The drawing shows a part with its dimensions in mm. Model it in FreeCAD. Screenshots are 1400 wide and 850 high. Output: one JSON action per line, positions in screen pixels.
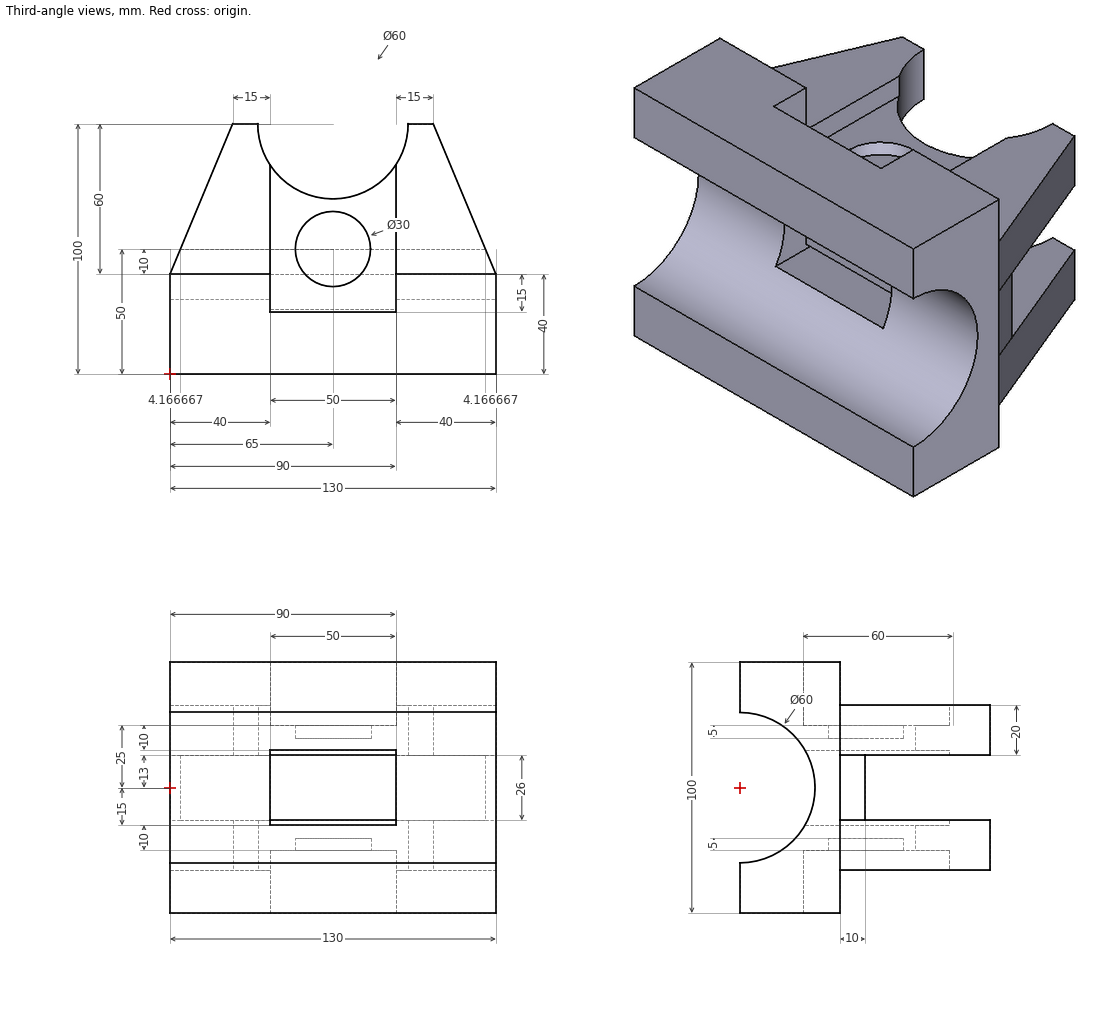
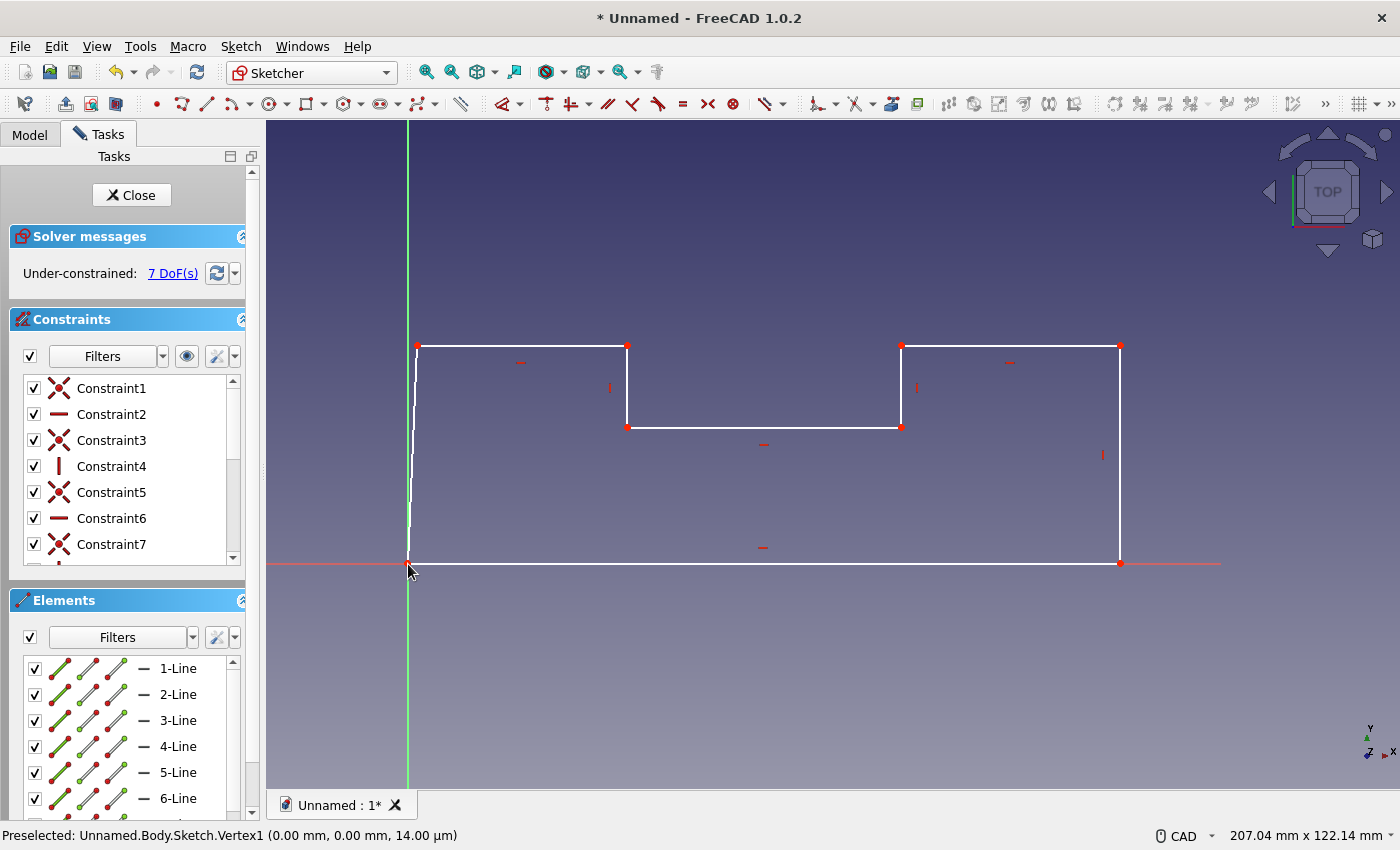
{"action": "left_click", "coordinate": [411, 499]}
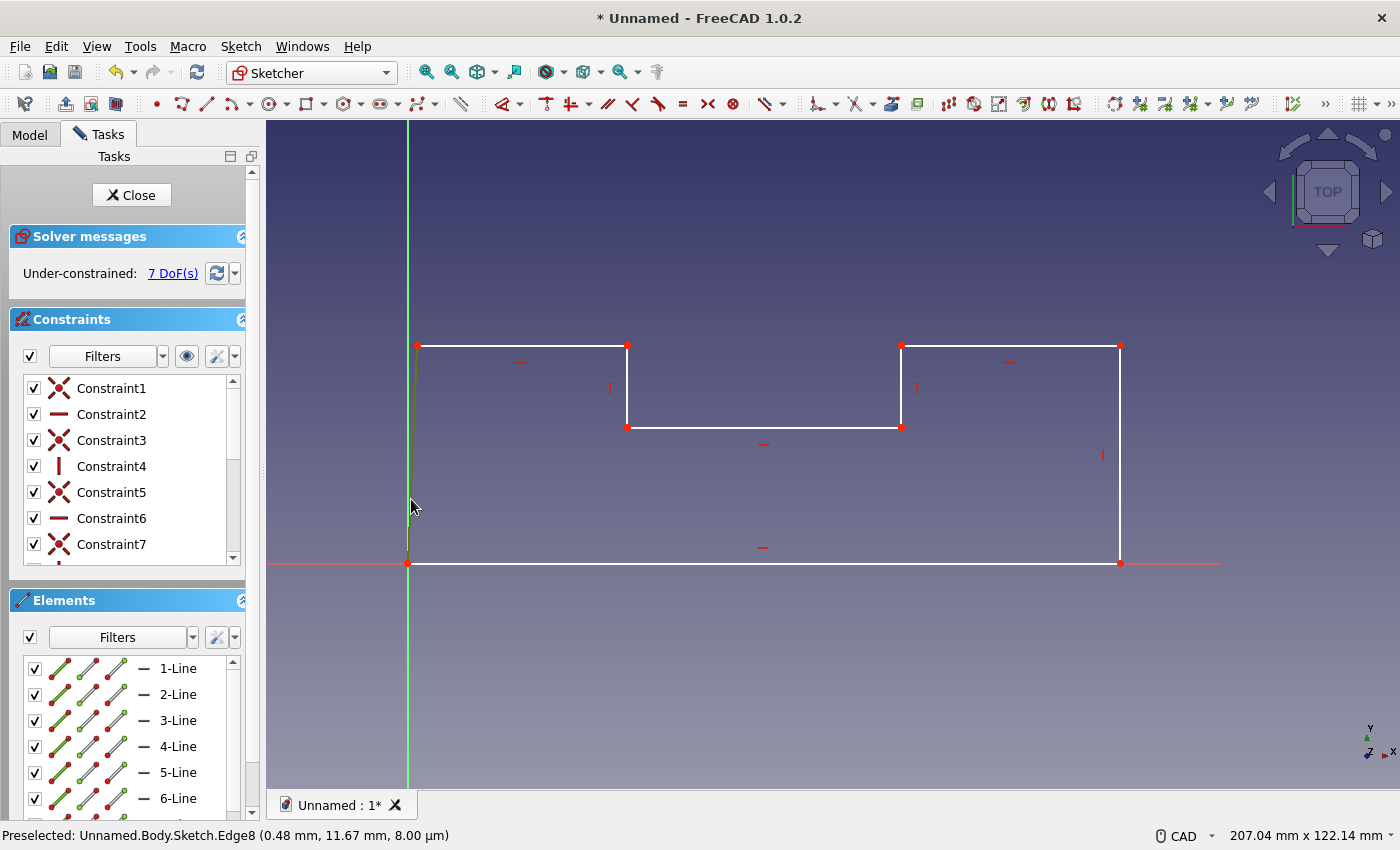
{"action": "key", "text": "v"}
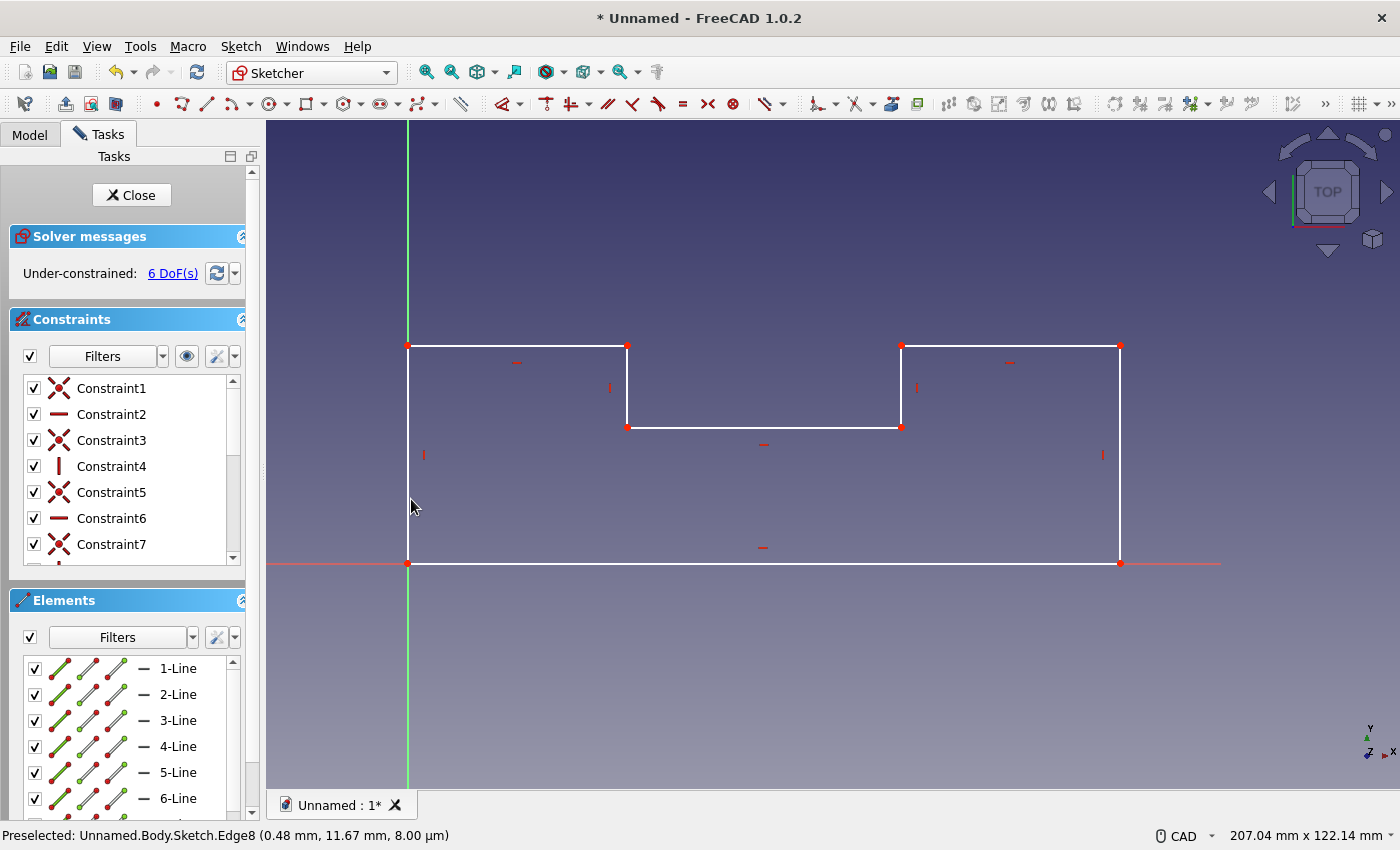
{"action": "left_click", "coordinate": [1120, 499]}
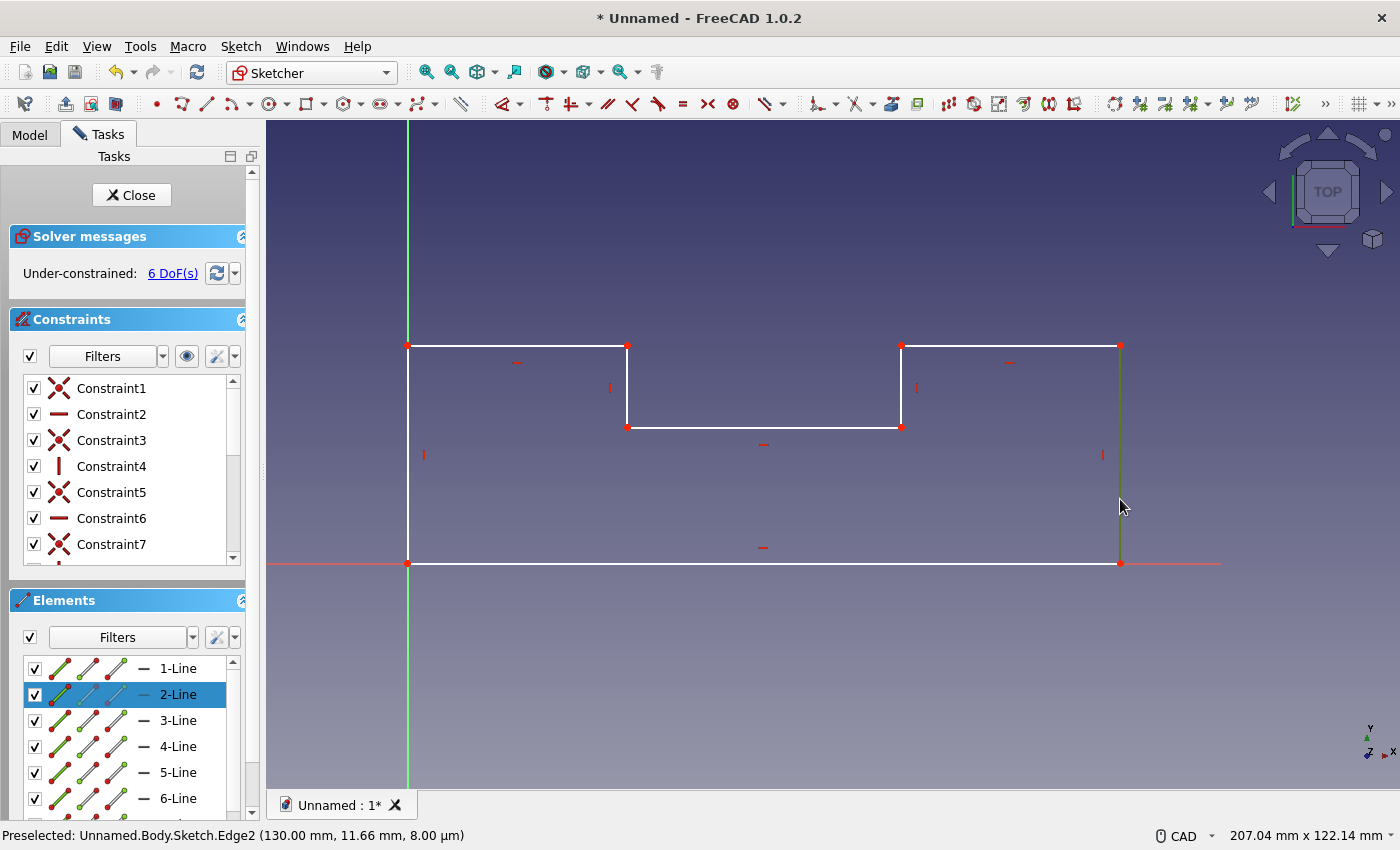
{"action": "key", "text": "i"}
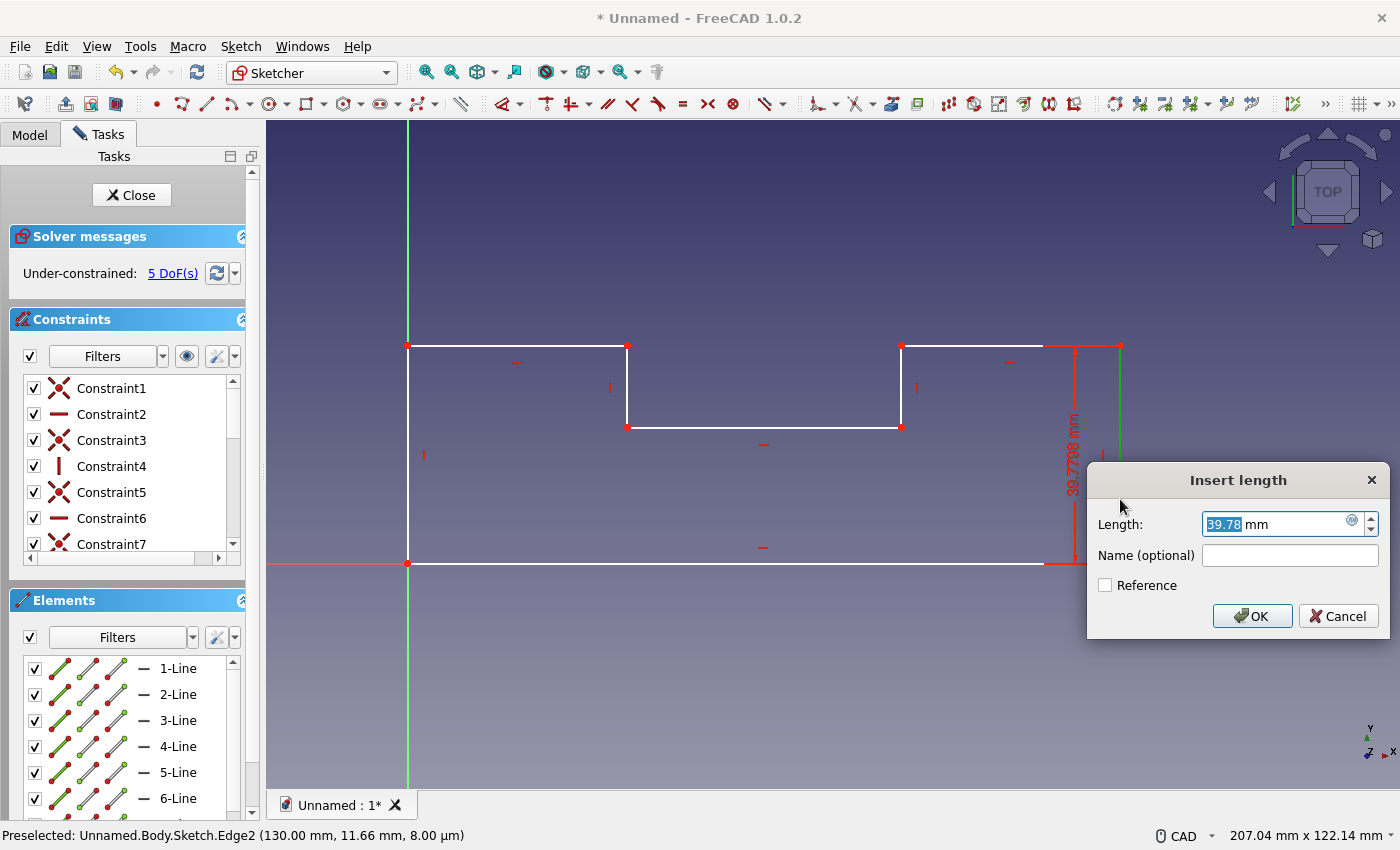
{"action": "type", "text": "40"}
{"action": "key", "text": "Return"}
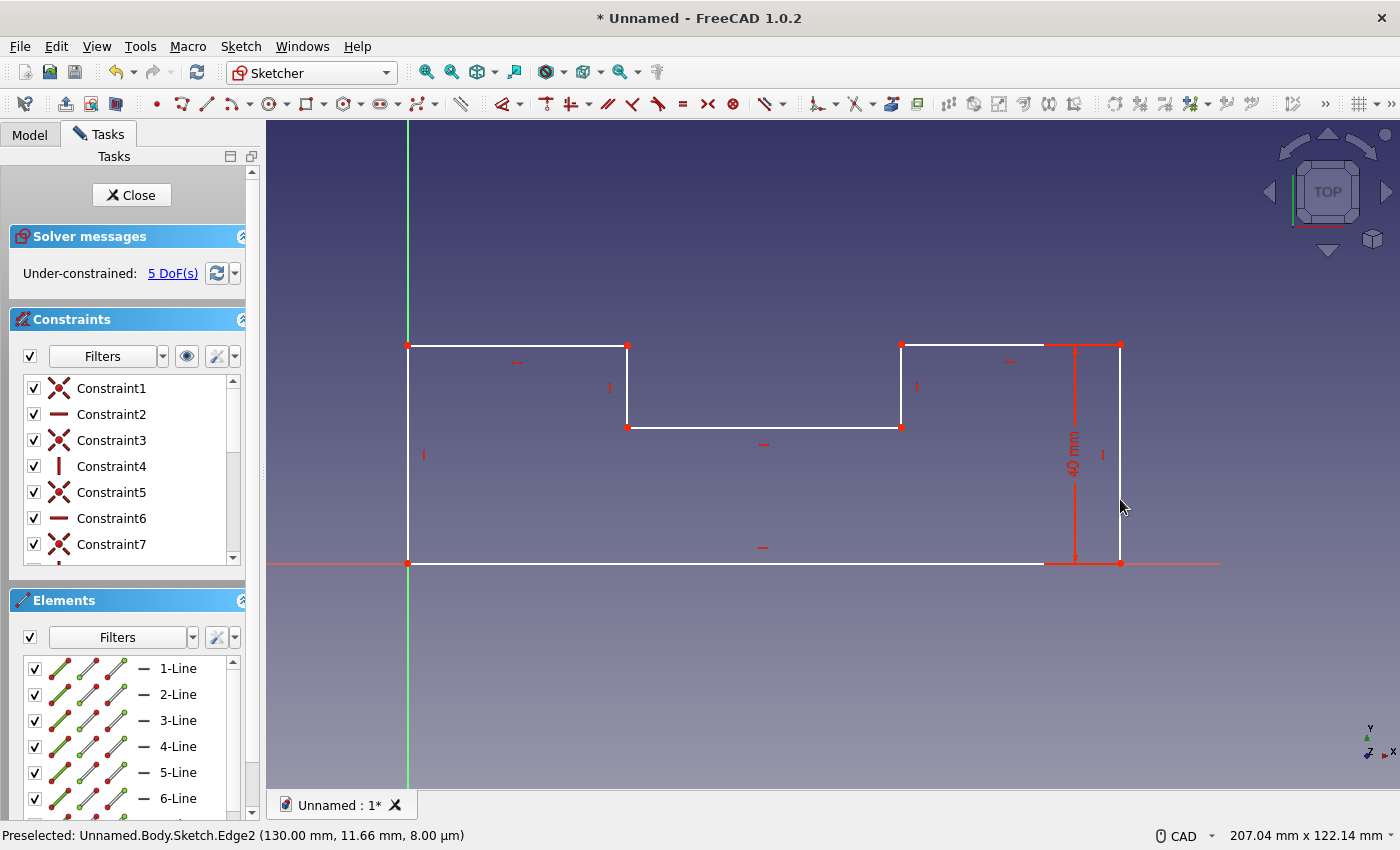
{"action": "left_click", "coordinate": [1054, 345]}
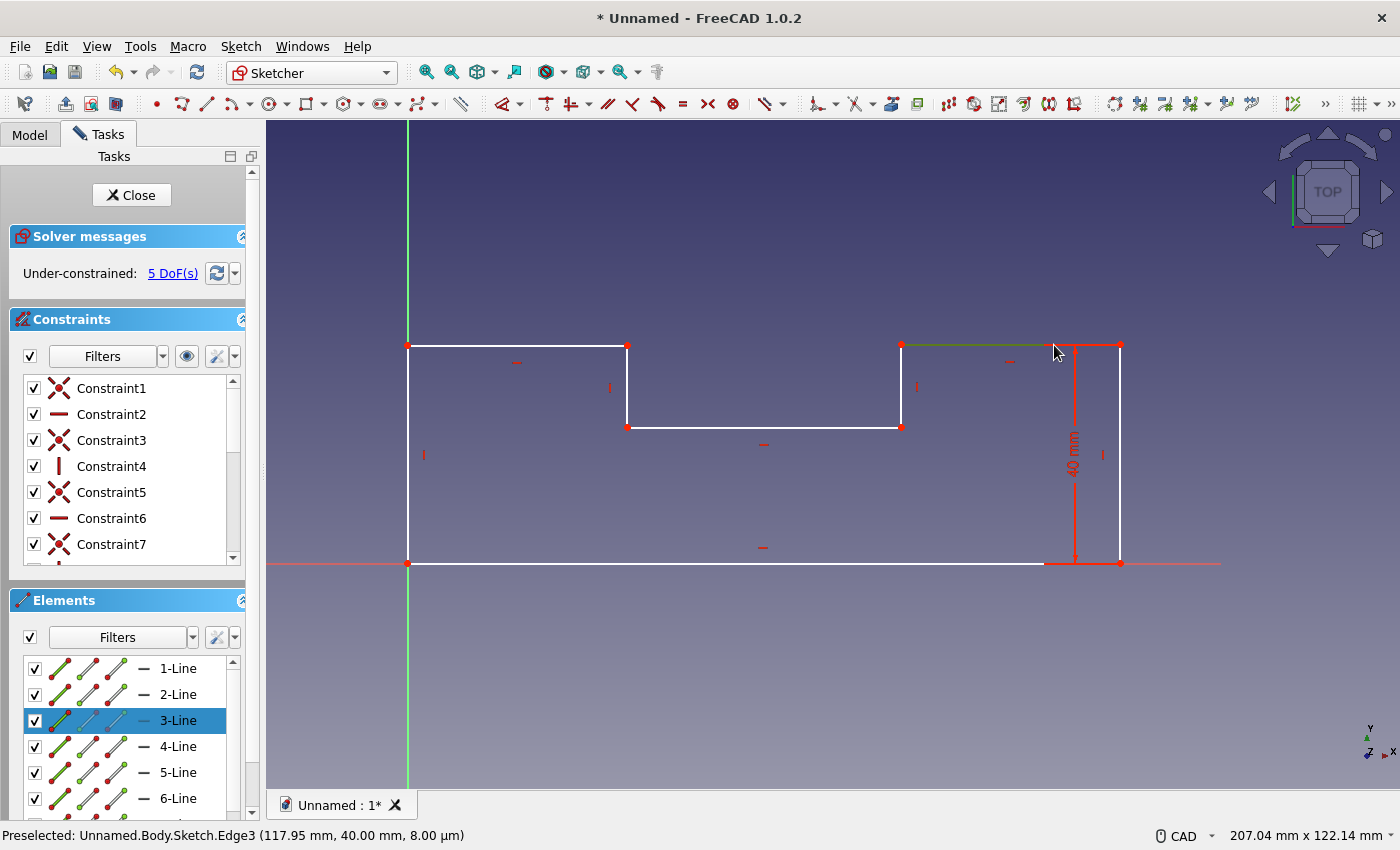
{"action": "key", "text": "l"}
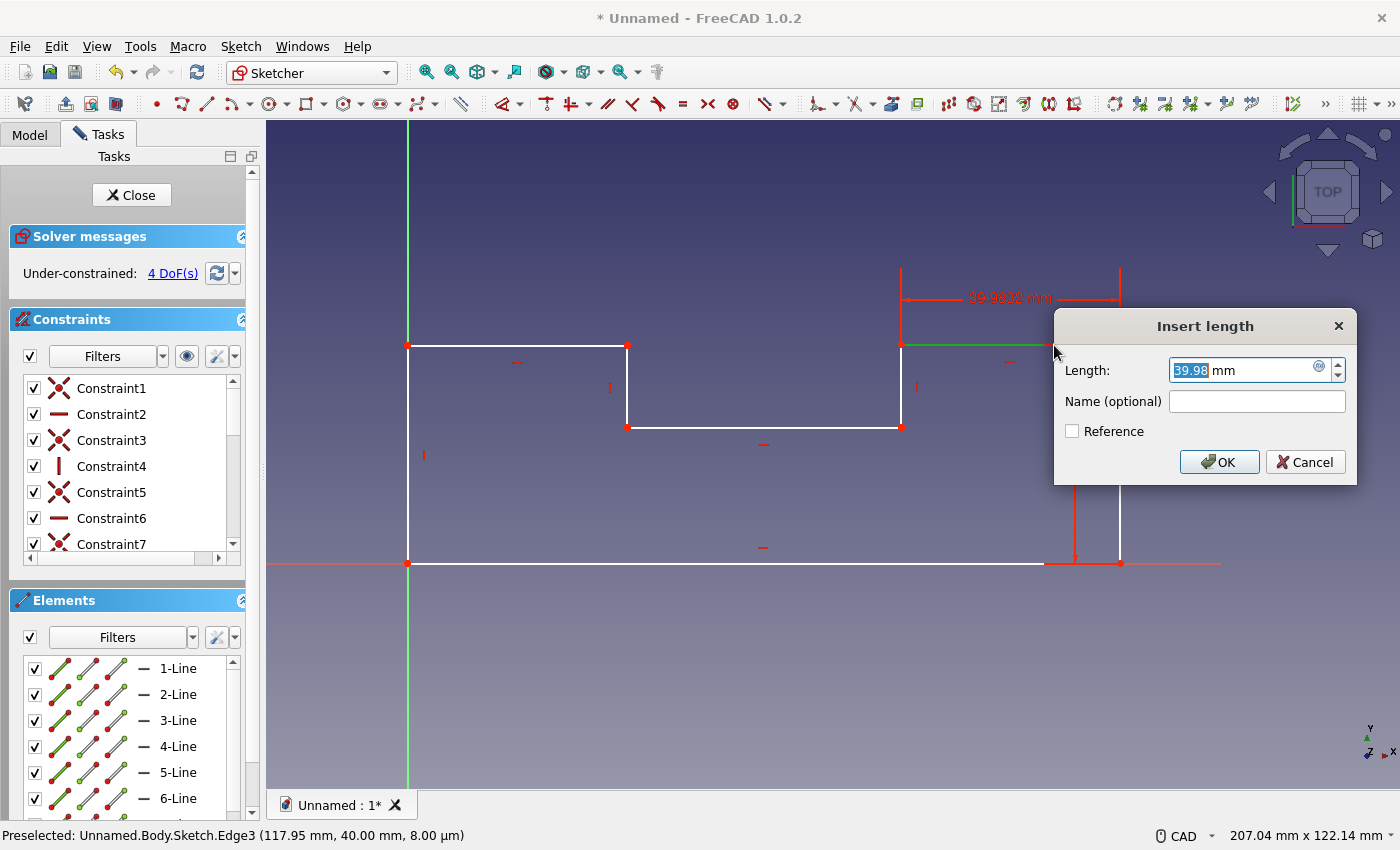
{"action": "type", "text": "40"}
{"action": "key", "text": "Return"}